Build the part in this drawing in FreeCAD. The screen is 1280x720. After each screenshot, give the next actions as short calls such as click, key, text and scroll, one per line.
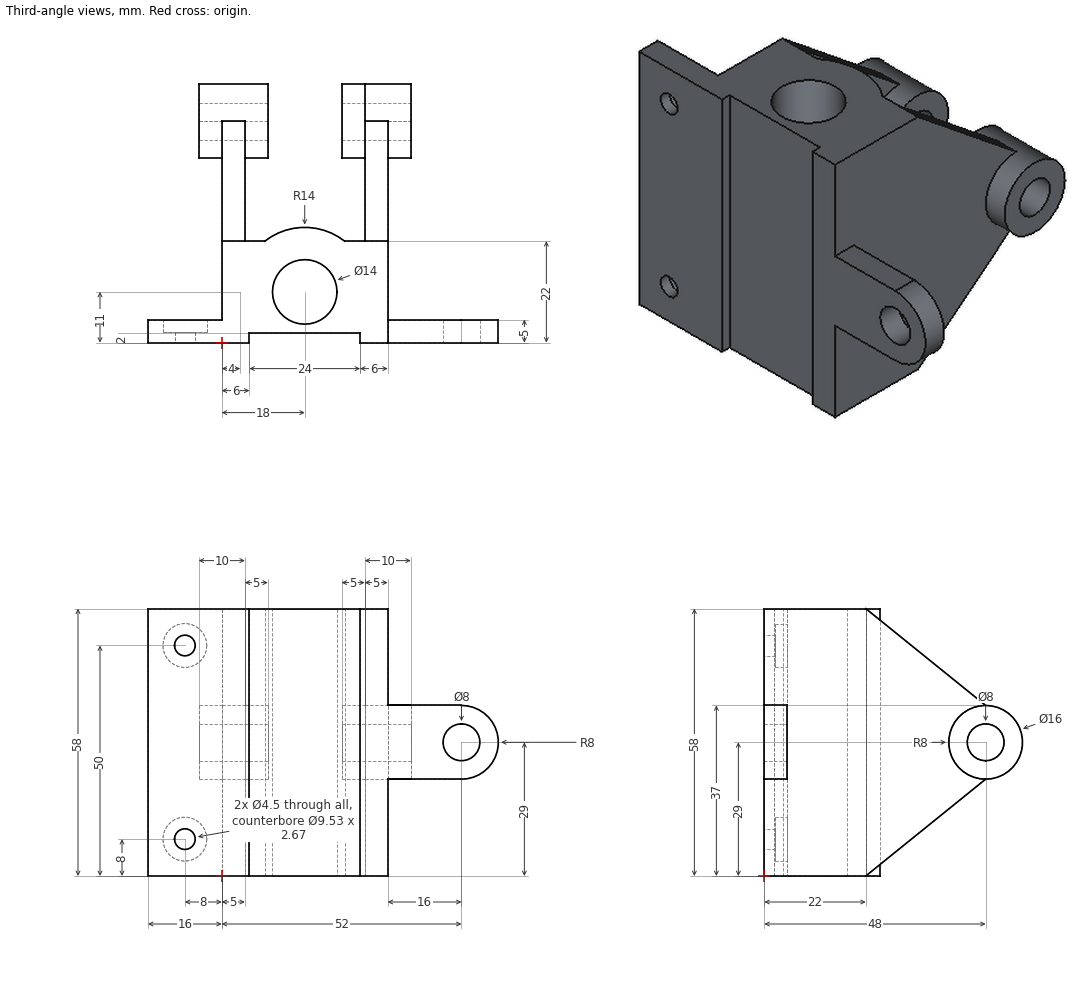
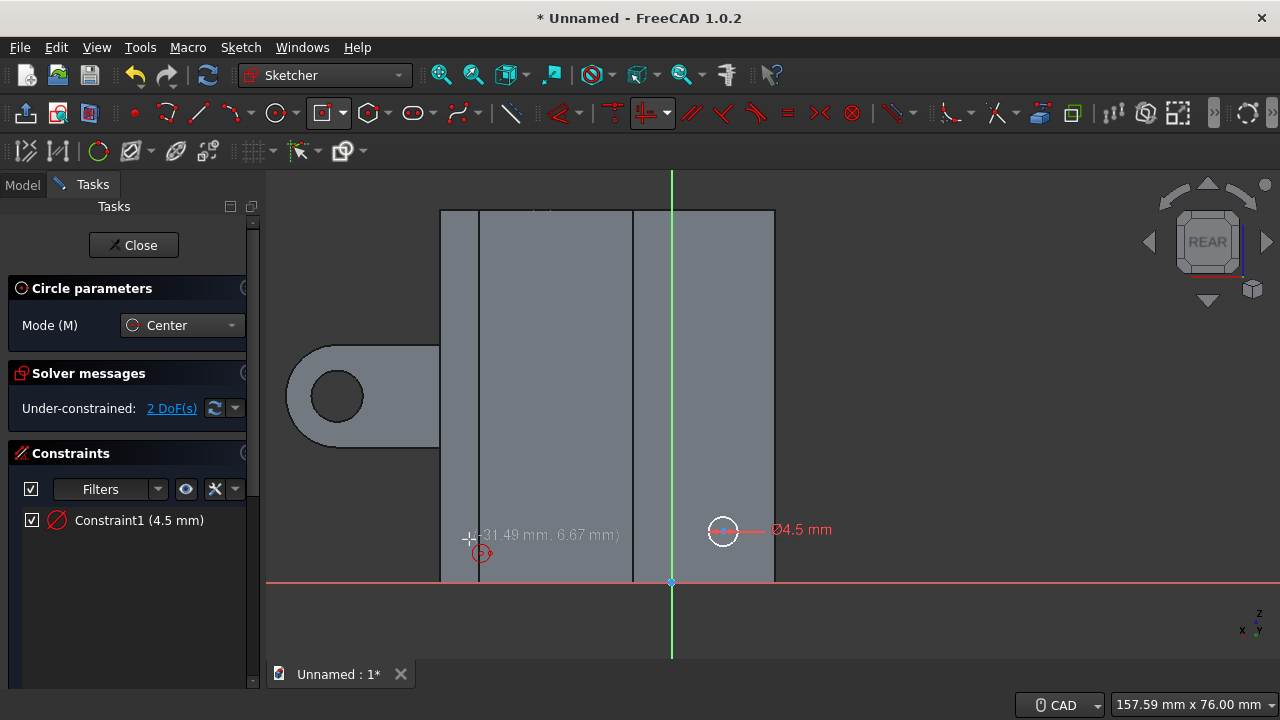
scroll(723, 261, up, 3)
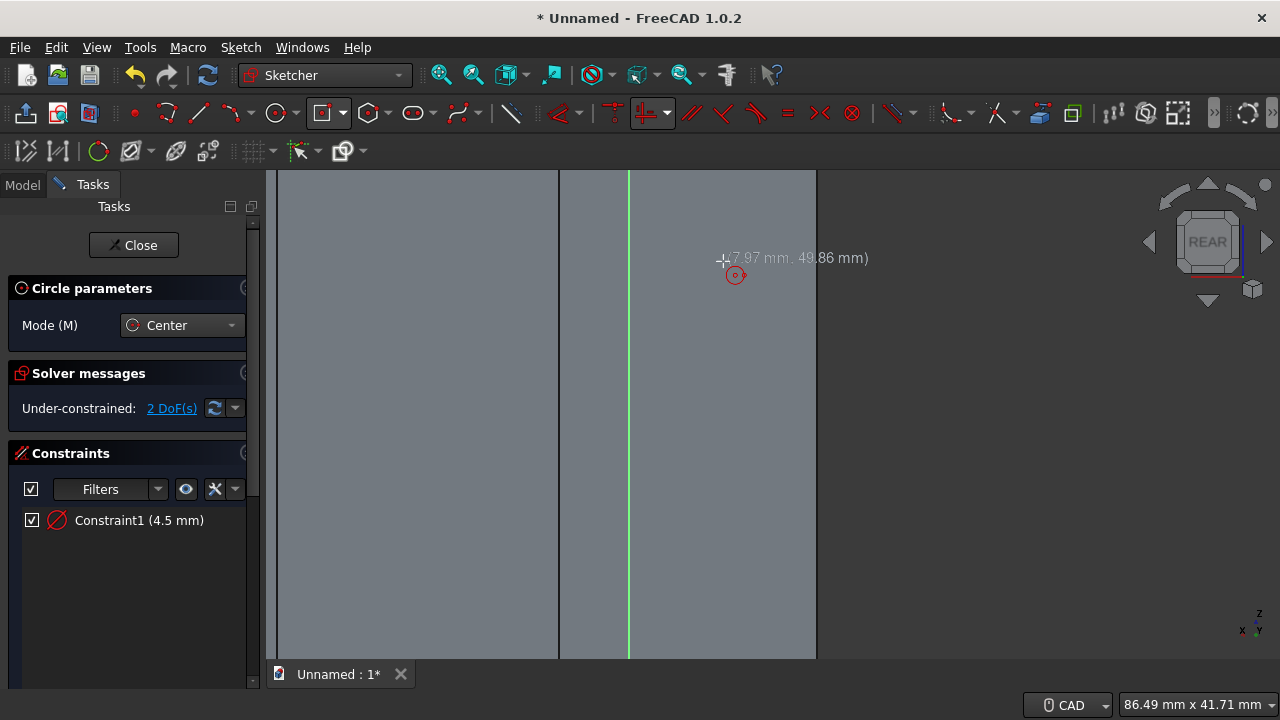
click(723, 261)
move(742, 242)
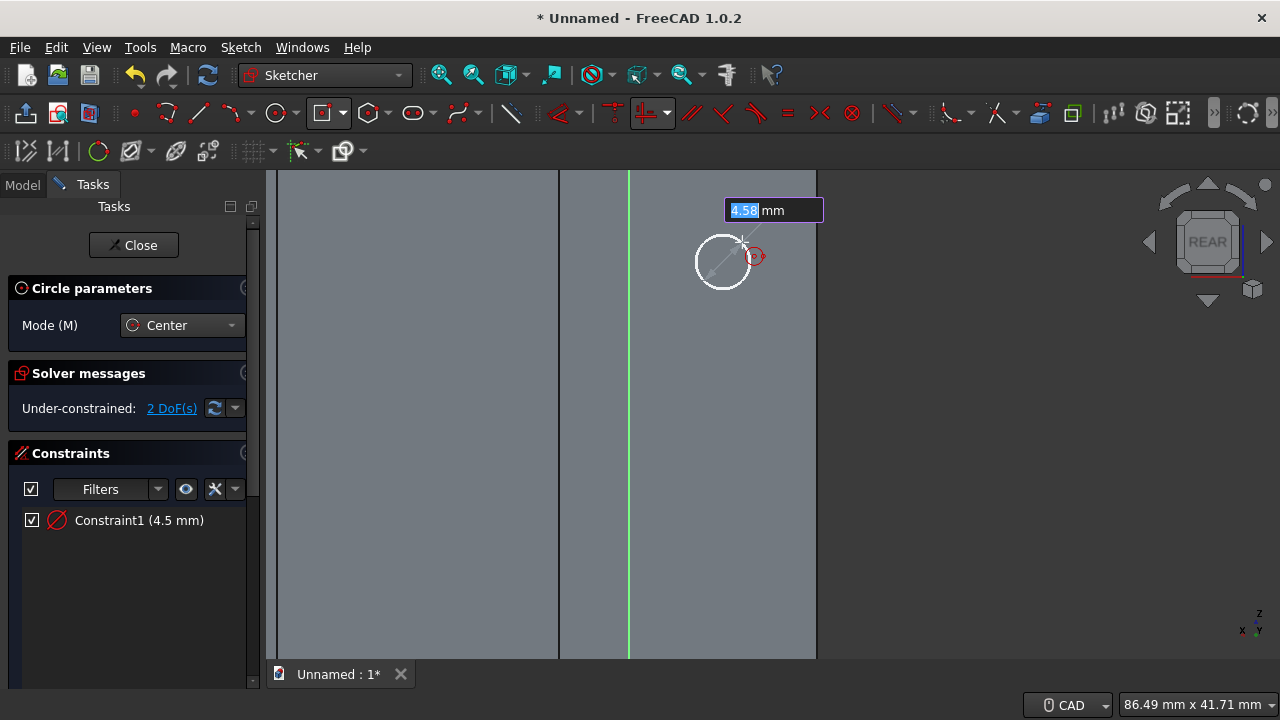
text(4.5)
key(Return)
key(Escape)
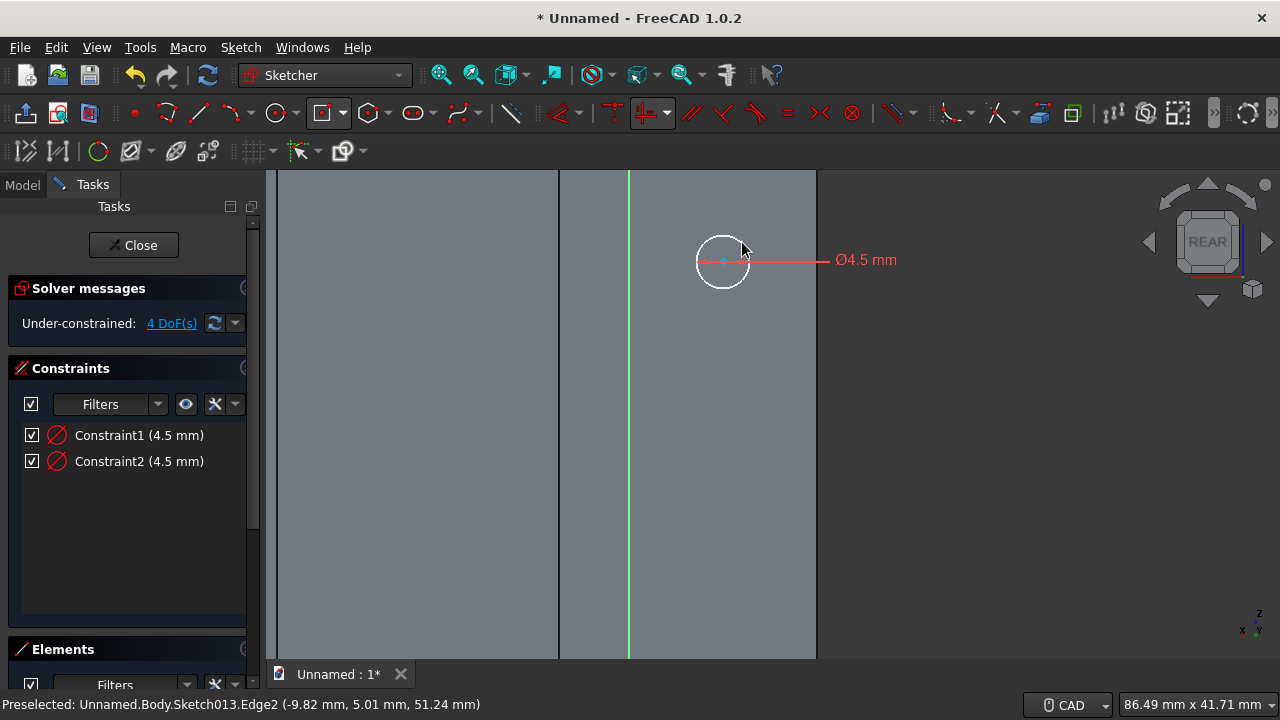
key(d)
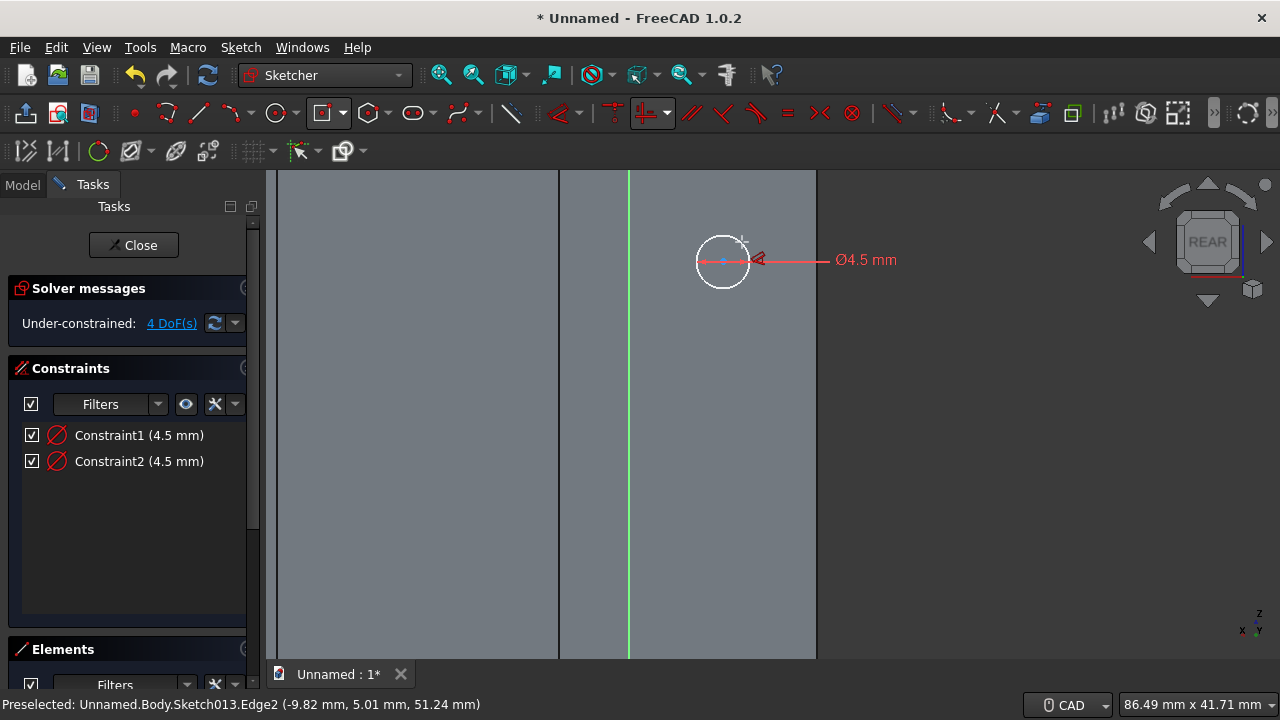
scroll(723, 261, down, 3)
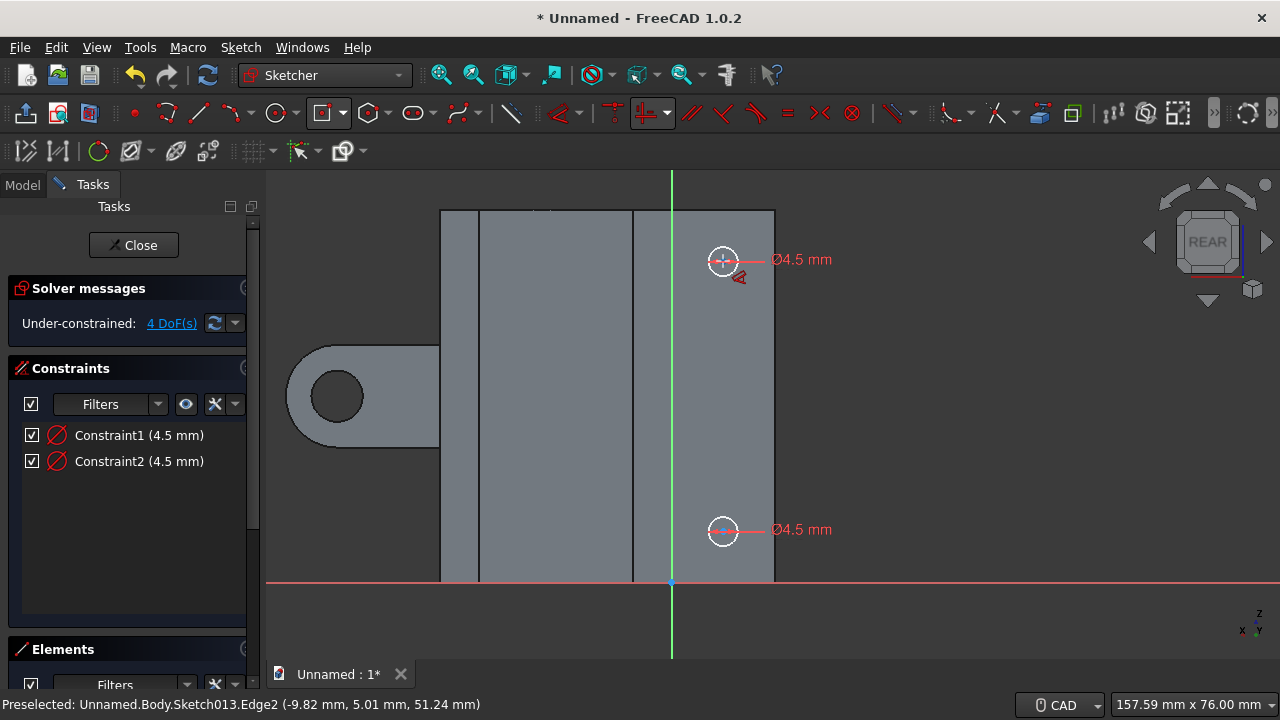
click(723, 532)
click(697, 617)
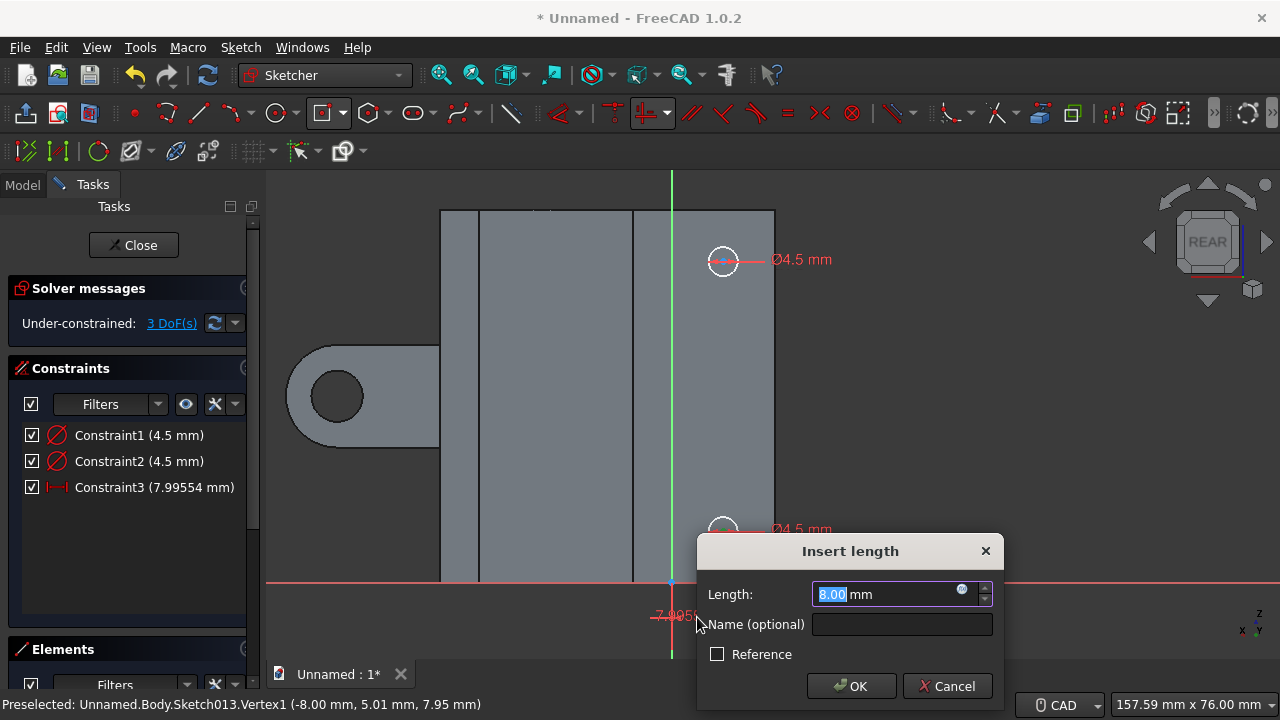
text(8)
key(Return)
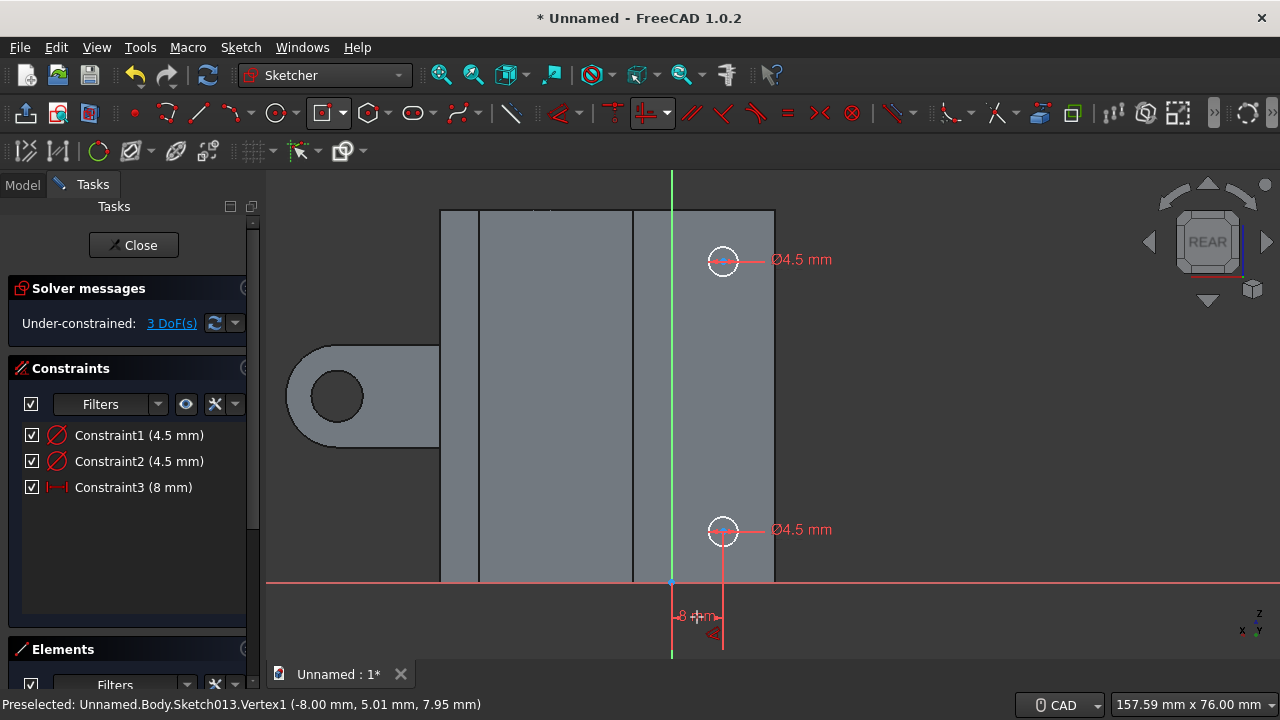
click(723, 532)
click(638, 557)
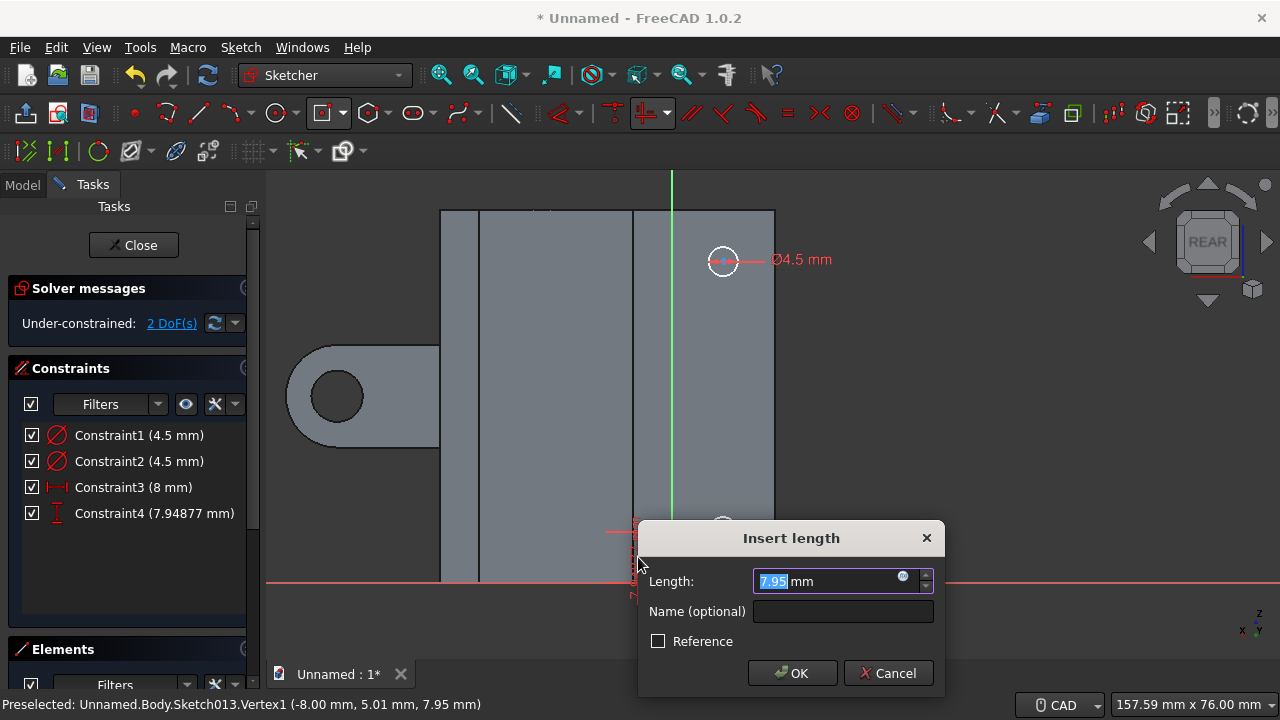
text(8)
key(Return)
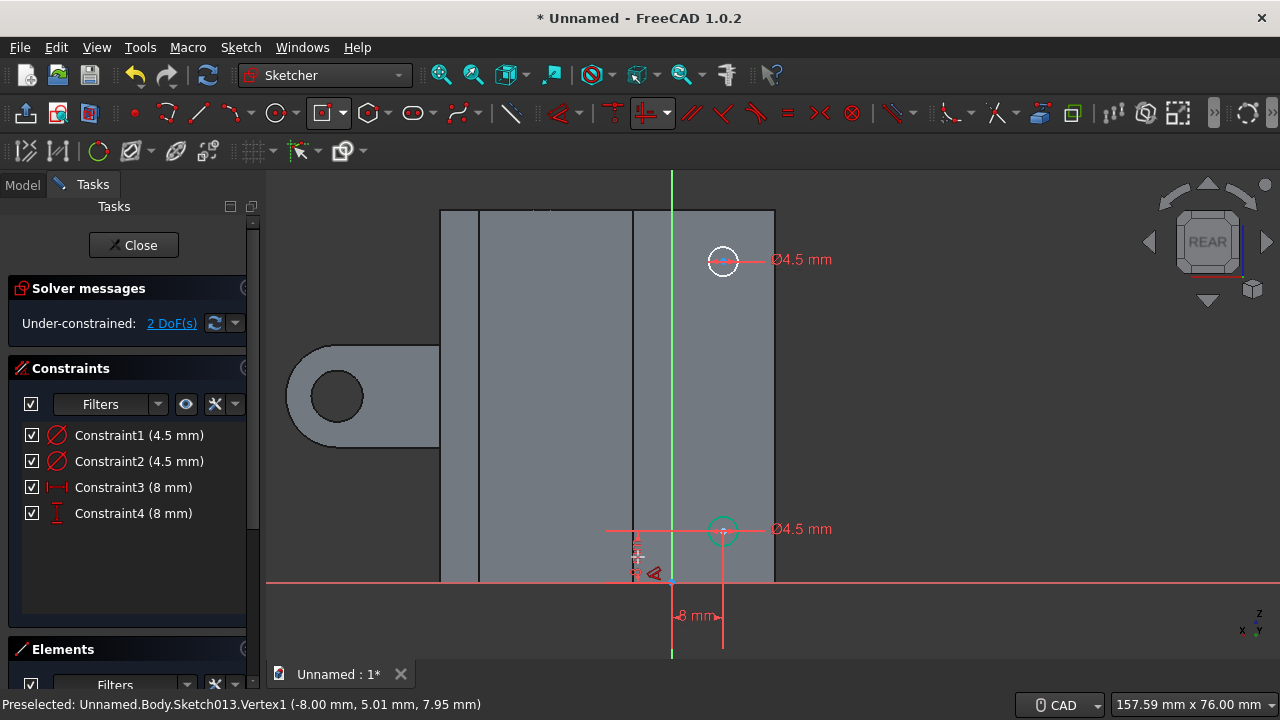
click(723, 262)
click(697, 228)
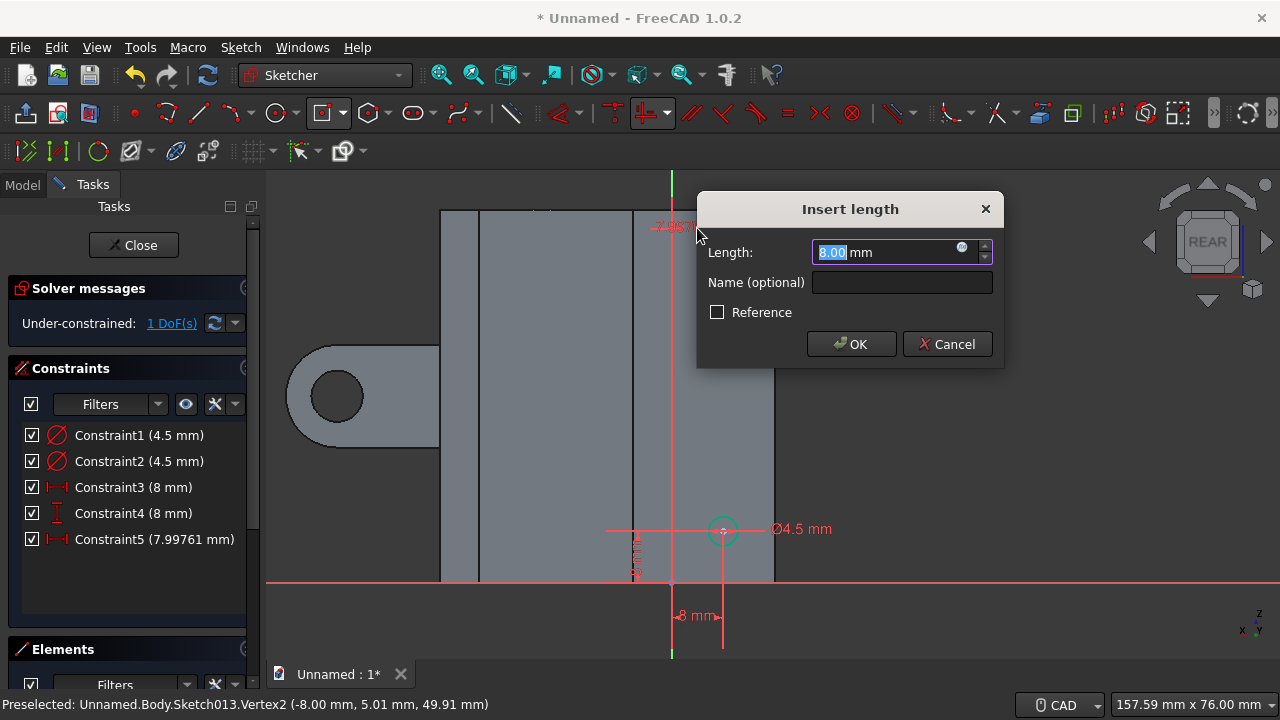
text(8)
key(Return)